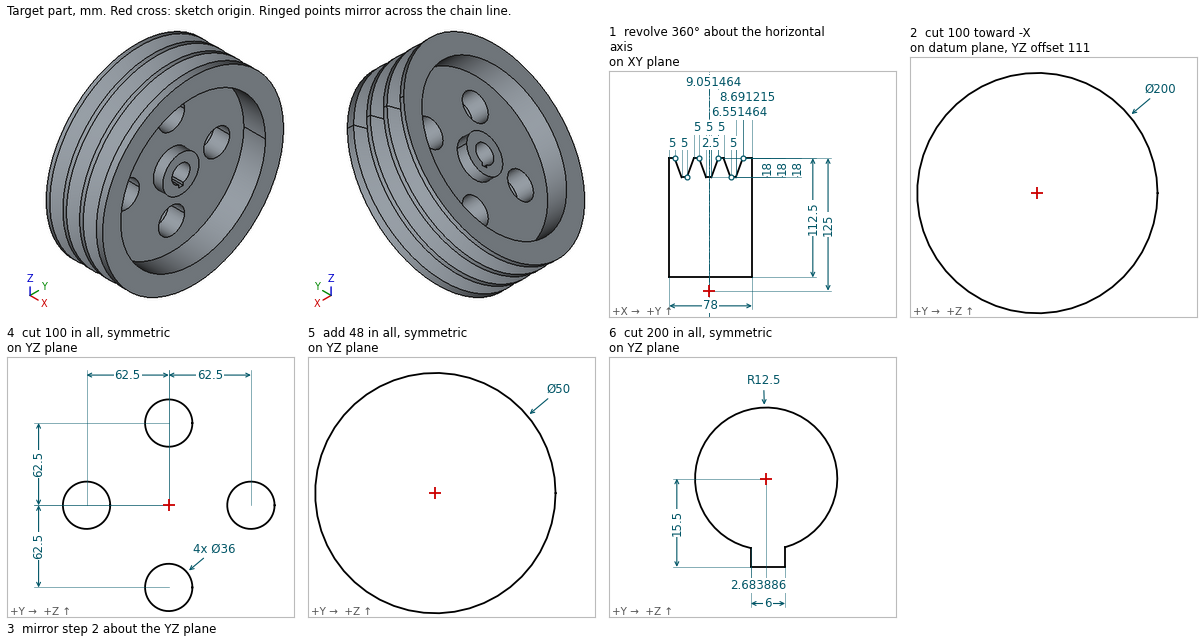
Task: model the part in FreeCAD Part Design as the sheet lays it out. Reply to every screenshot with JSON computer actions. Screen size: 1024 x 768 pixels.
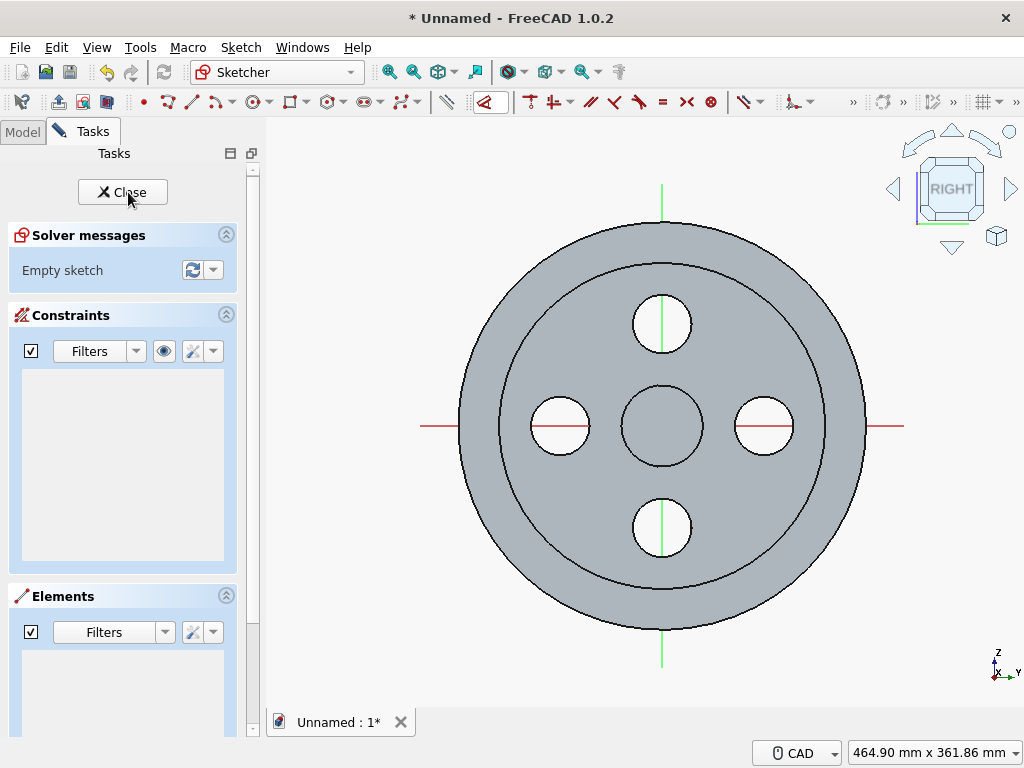
{"action": "left_click", "coordinate": [108, 102]}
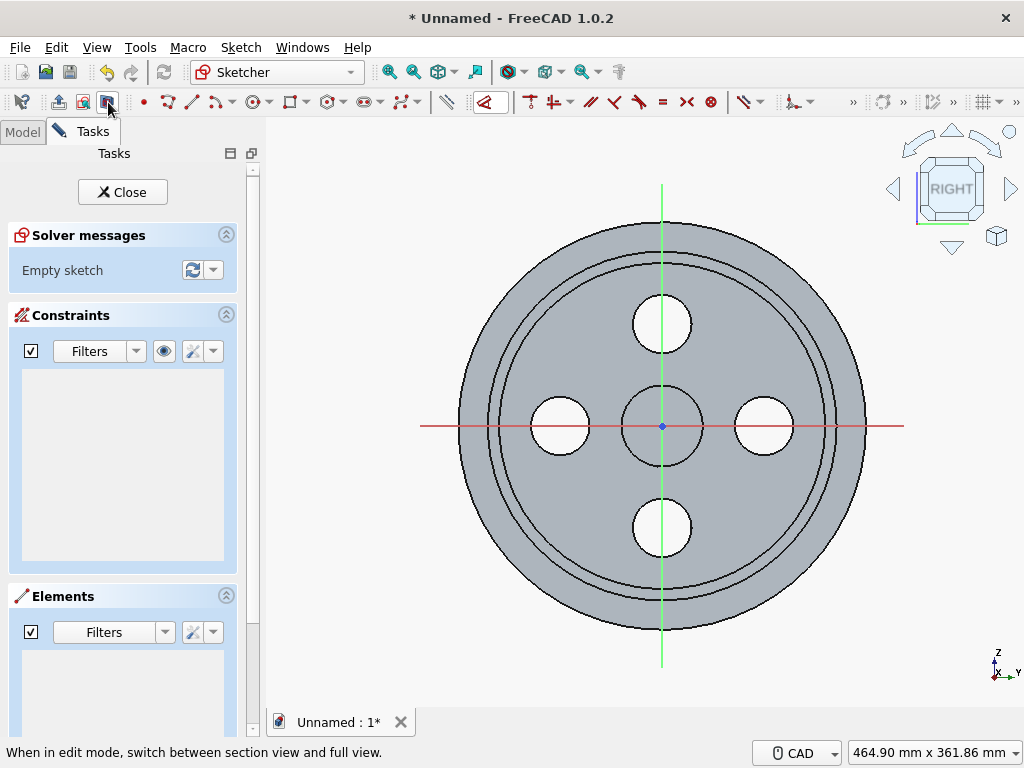
{"action": "scroll", "coordinate": [673, 431], "scroll_direction": "up", "scroll_amount": 11}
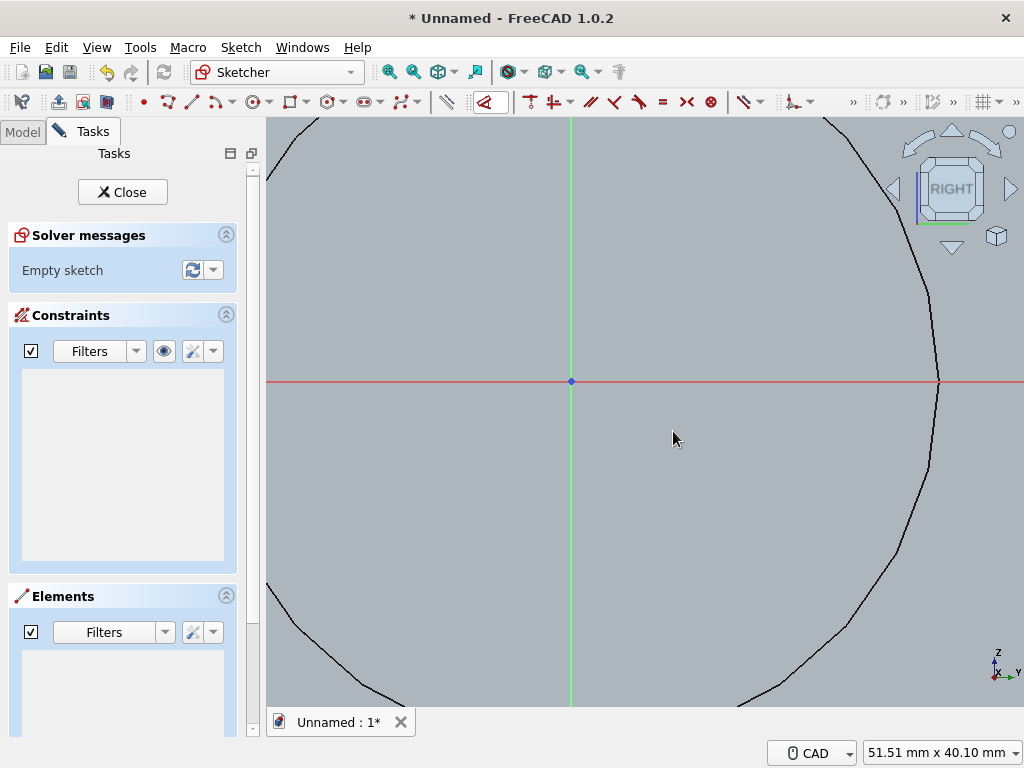
{"action": "left_click", "coordinate": [168, 102]}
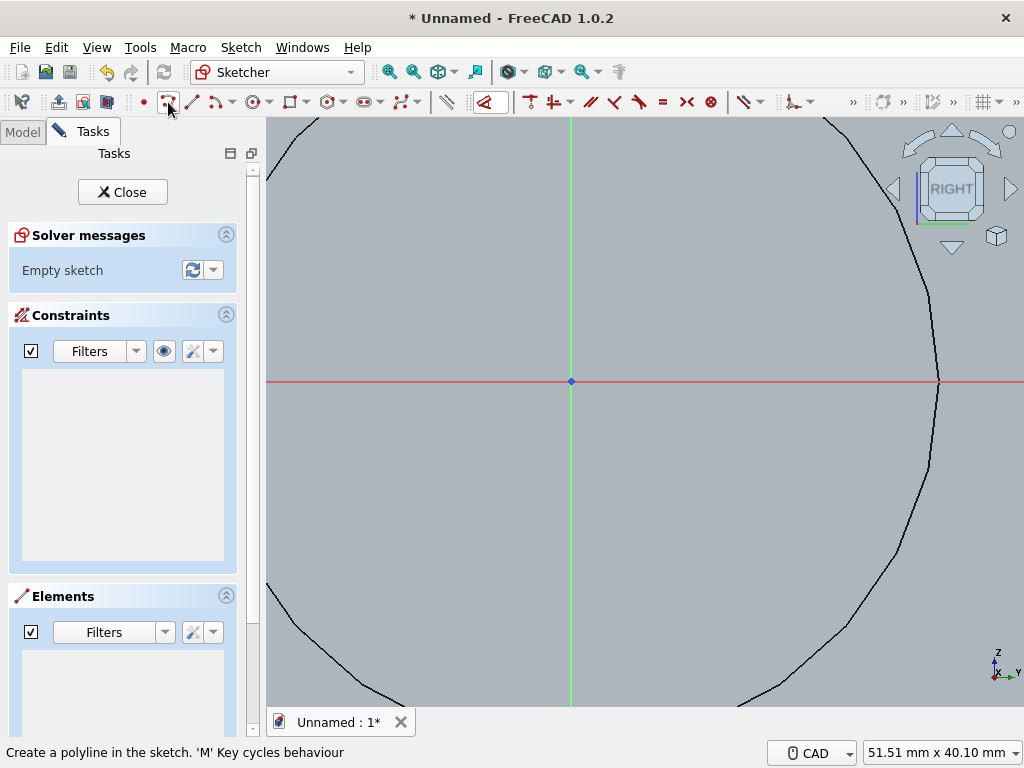
{"action": "left_click", "coordinate": [532, 561]}
{"action": "left_click", "coordinate": [532, 610]}
{"action": "left_click", "coordinate": [620, 610]}
{"action": "left_click", "coordinate": [620, 559]}
{"action": "right_click", "coordinate": [620, 559]}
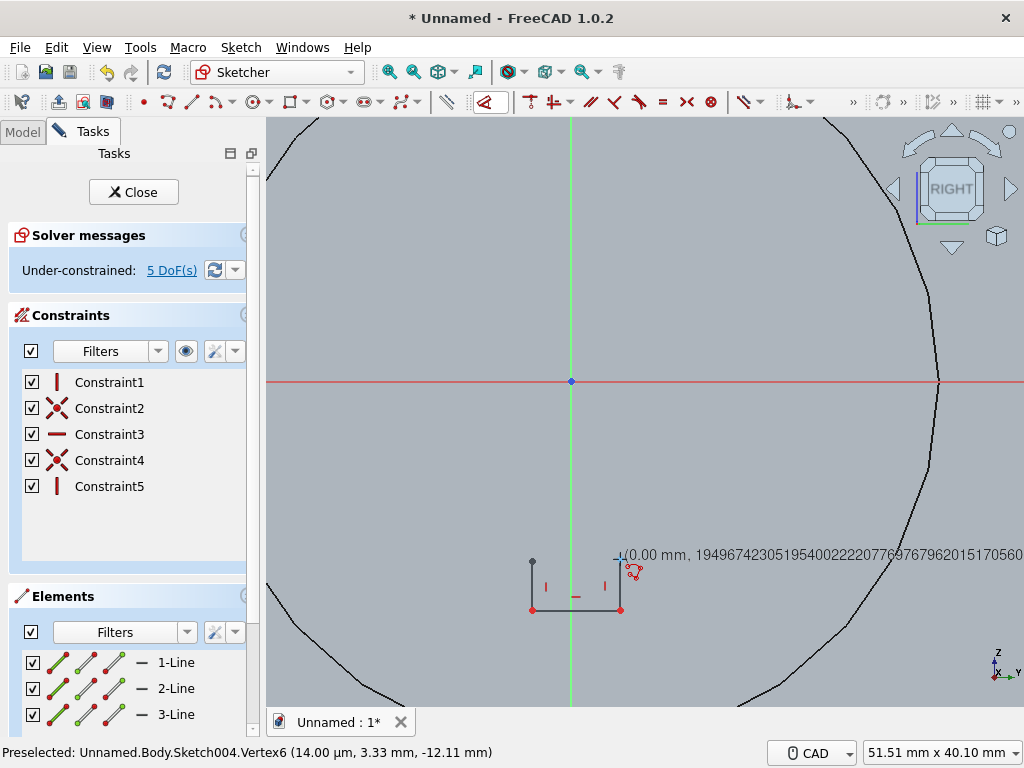
{"action": "left_click", "coordinate": [234, 102]}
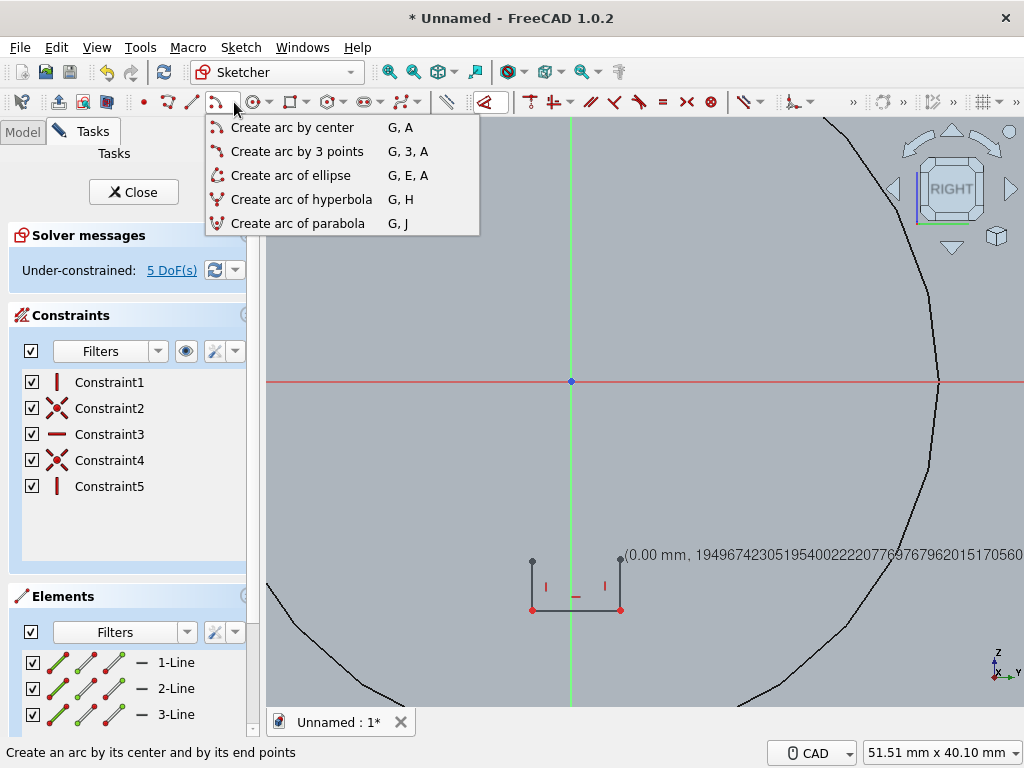
{"action": "left_click", "coordinate": [342, 151]}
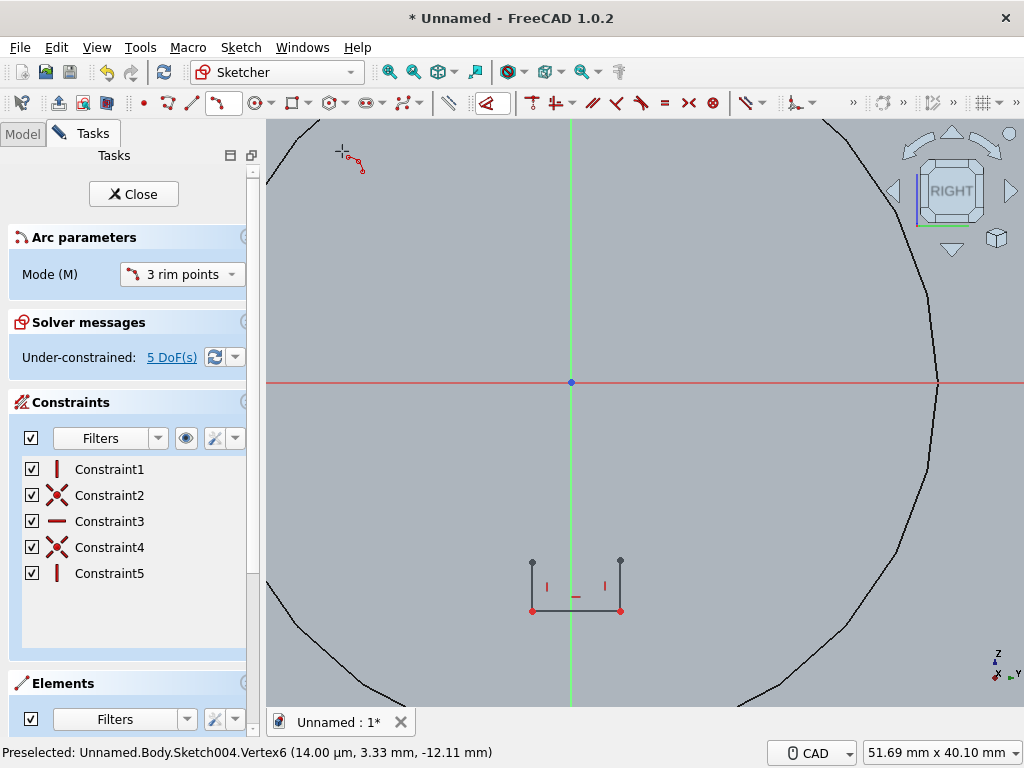
{"action": "left_click", "coordinate": [620, 560]}
{"action": "left_click", "coordinate": [532, 562]}
{"action": "left_click", "coordinate": [668, 227]}
{"action": "key", "text": "Escape"}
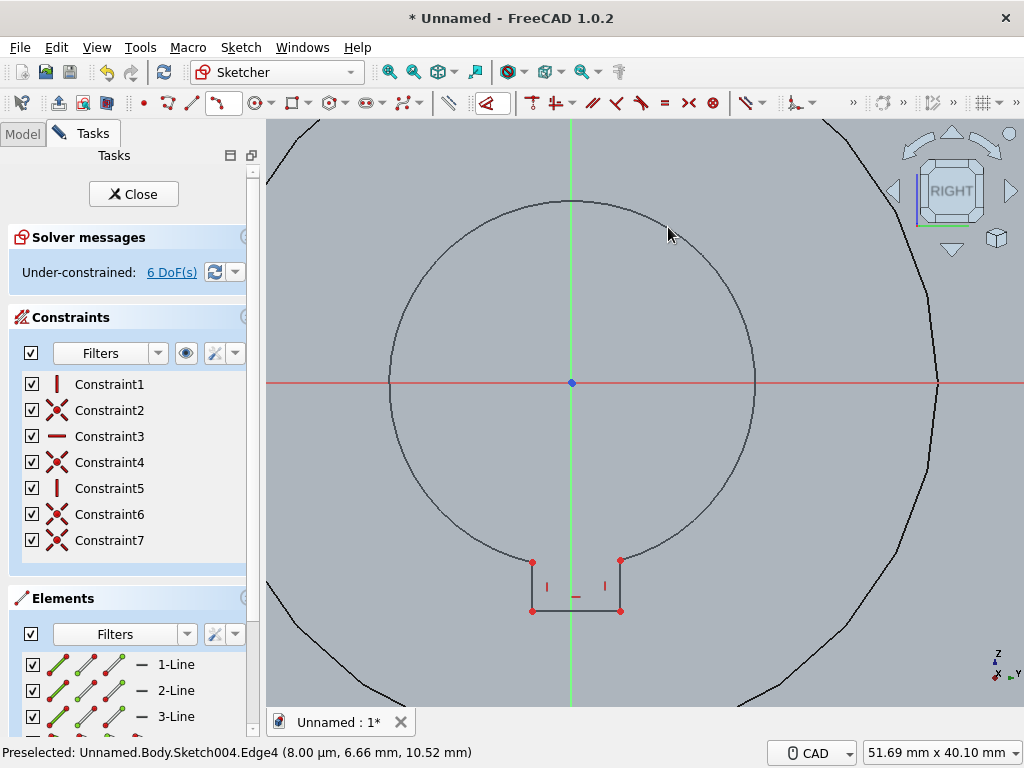
{"action": "left_click_drag", "start_coordinate": [561, 373], "coordinate": [582, 394]}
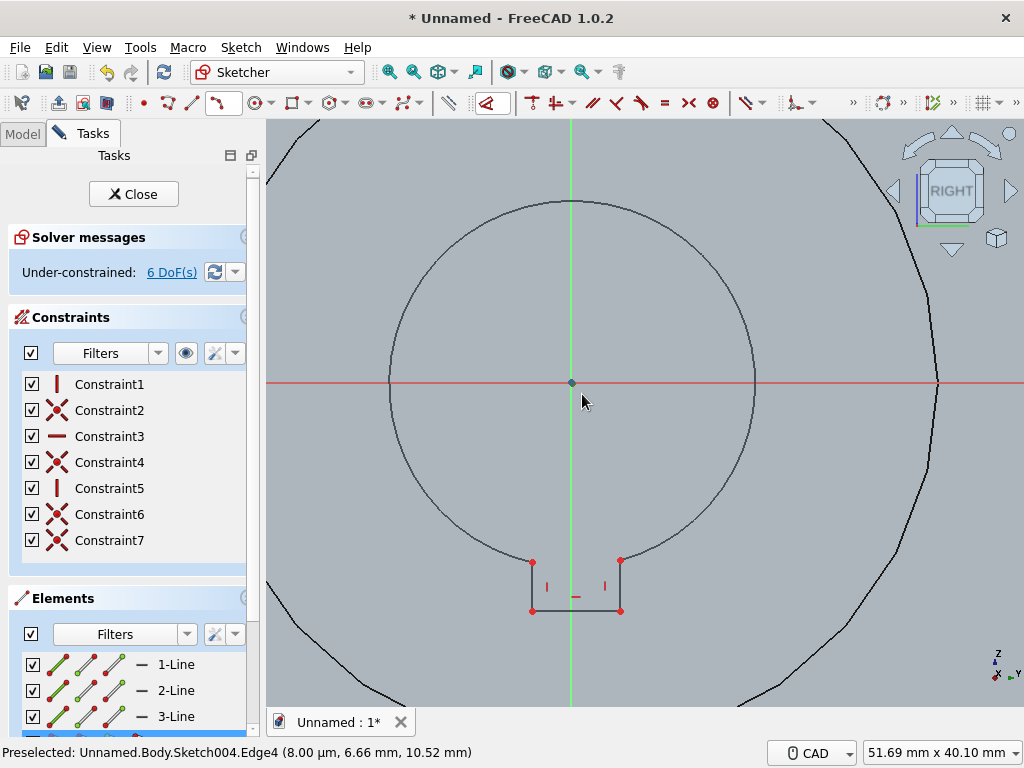
{"action": "left_click", "coordinate": [532, 104]}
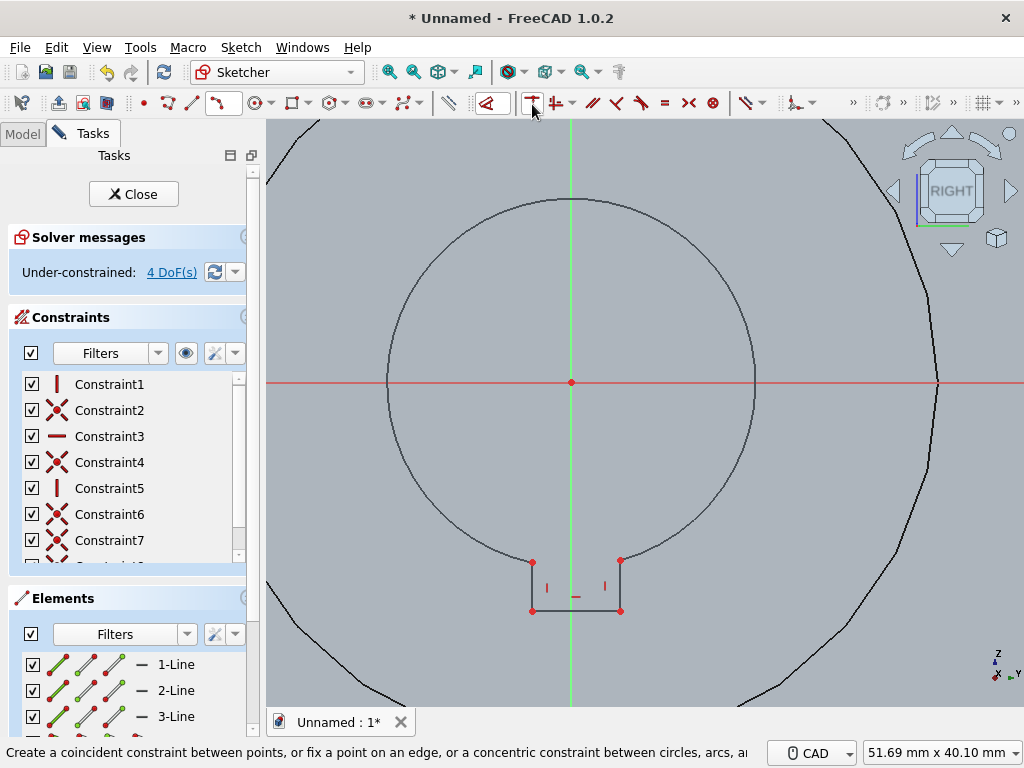
{"action": "left_click", "coordinate": [738, 305]}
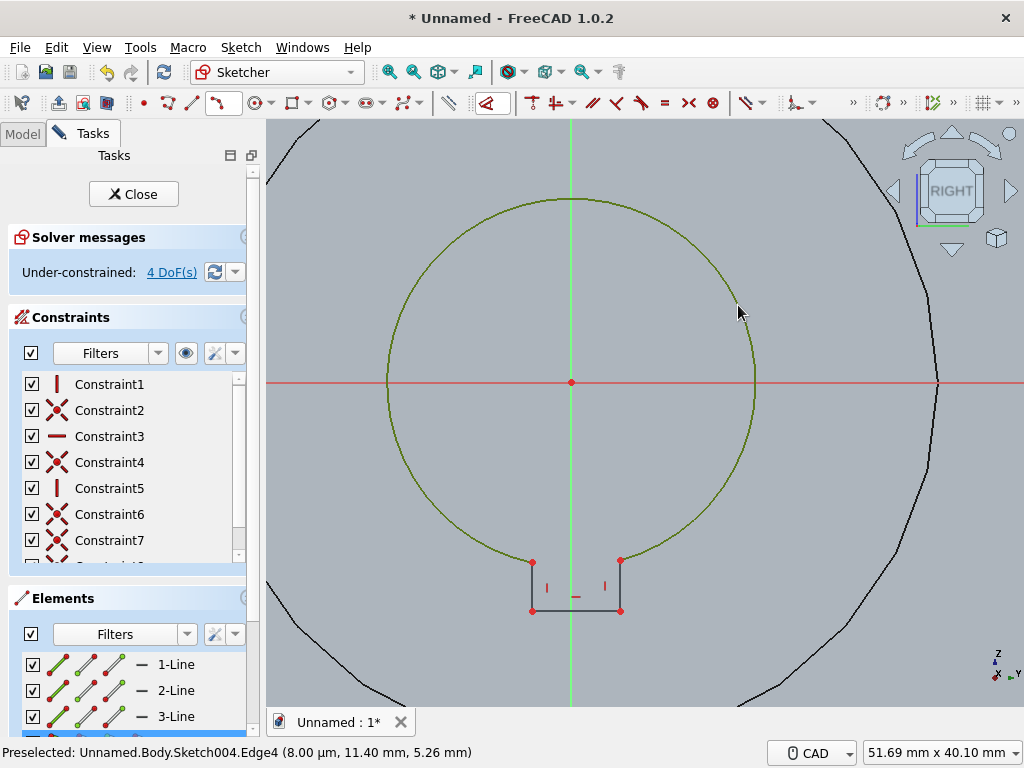
{"action": "left_click", "coordinate": [504, 104]}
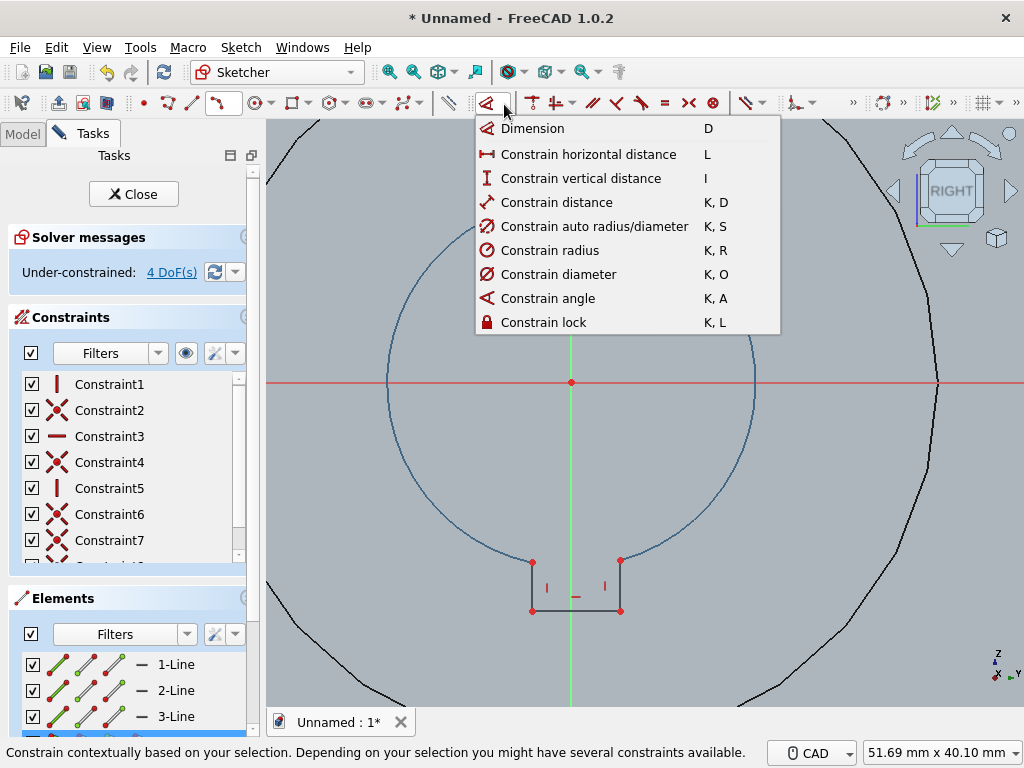
{"action": "left_click", "coordinate": [628, 250]}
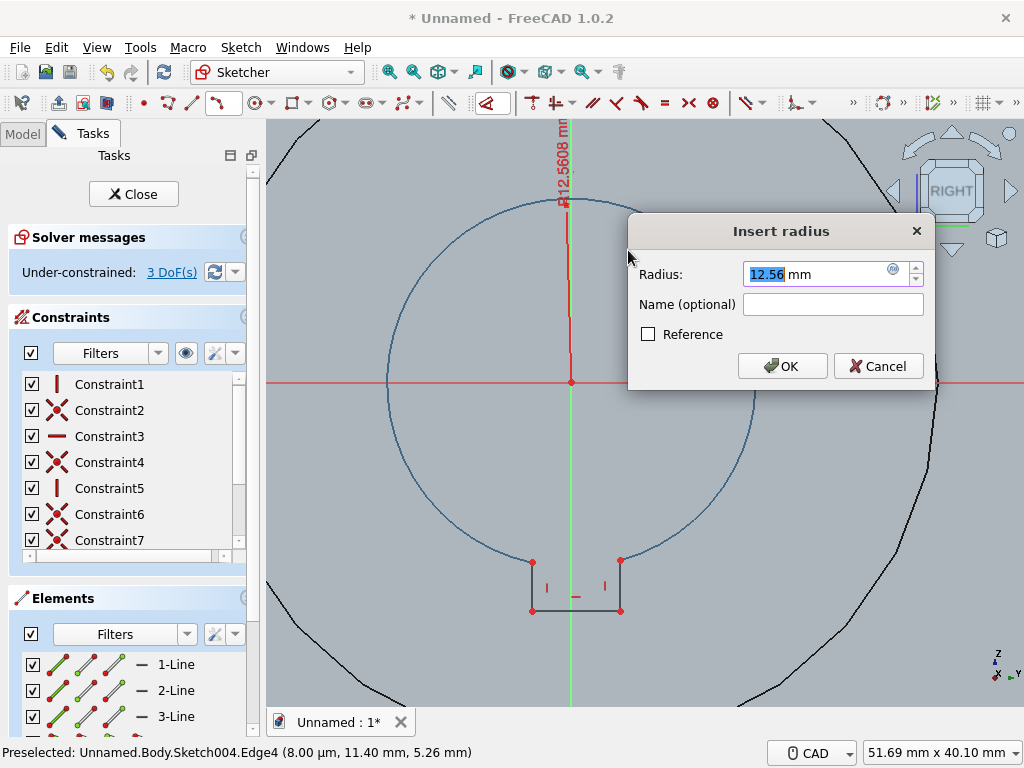
{"action": "type", "text": "12.5"}
{"action": "key", "text": "Return"}